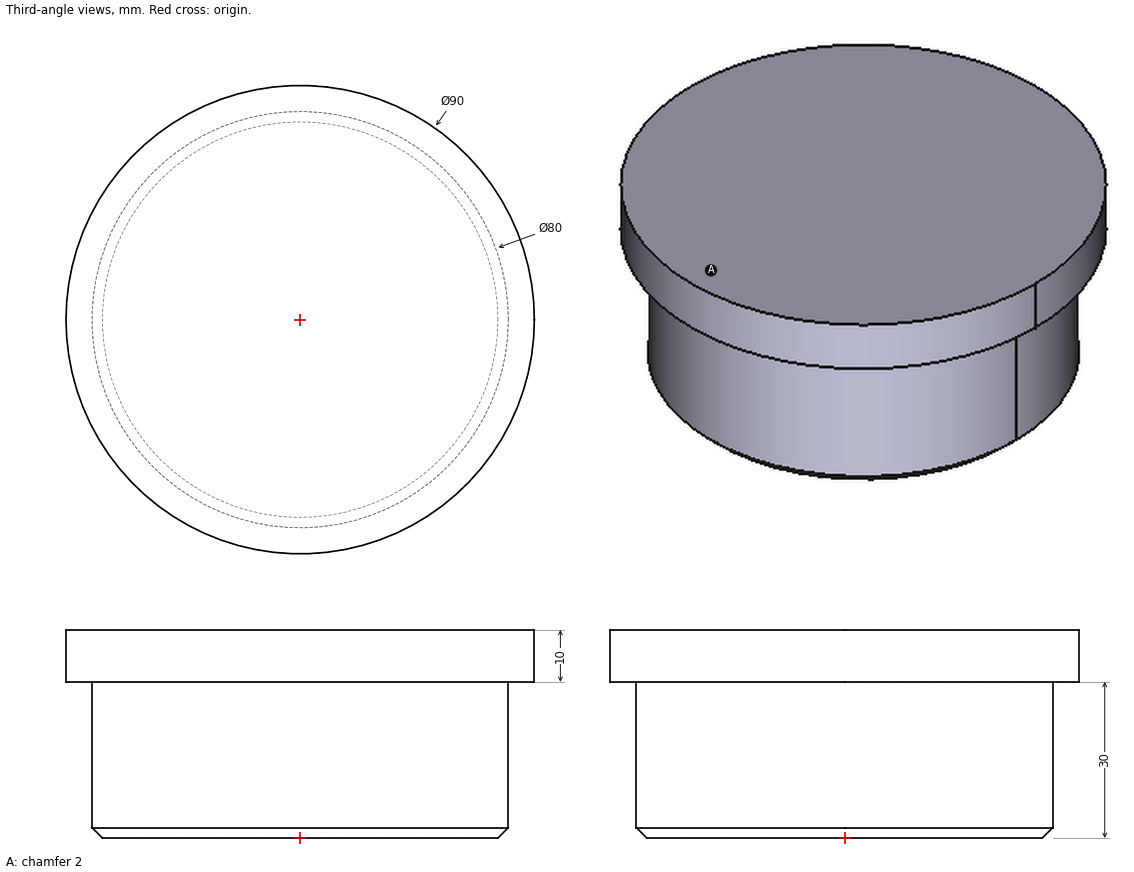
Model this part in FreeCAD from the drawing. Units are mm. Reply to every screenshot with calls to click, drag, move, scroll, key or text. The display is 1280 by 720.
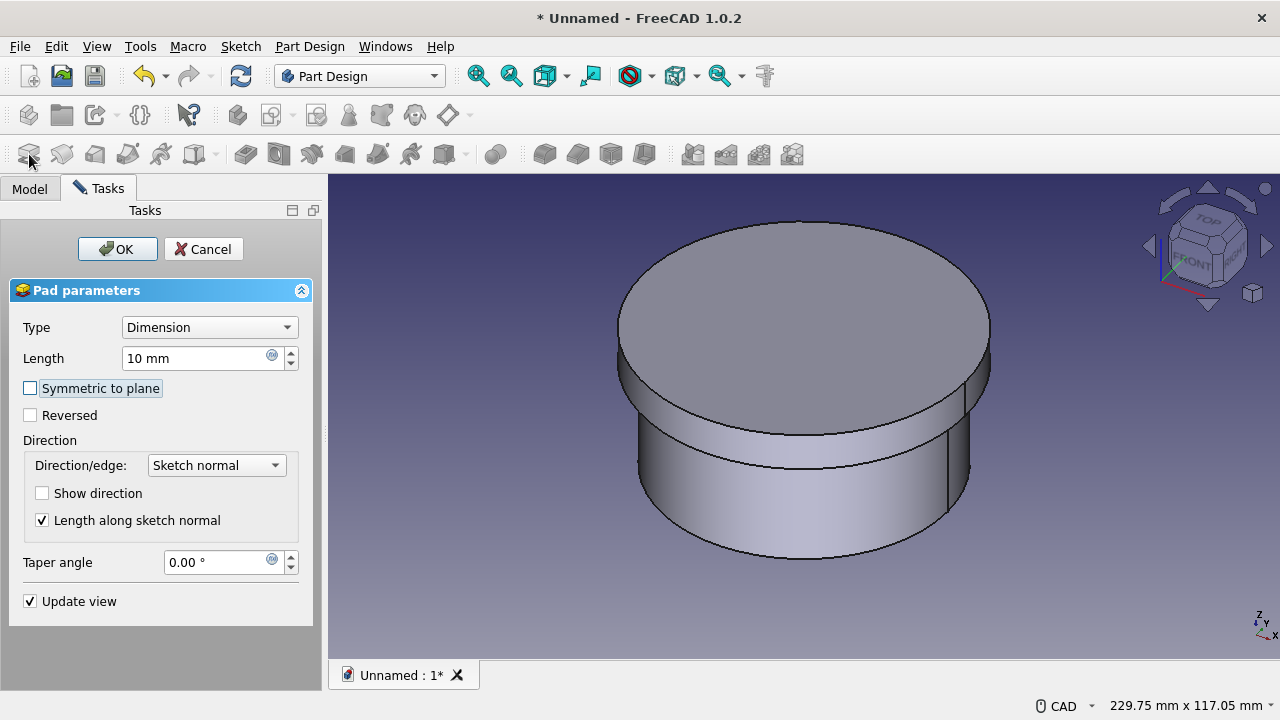
click(118, 249)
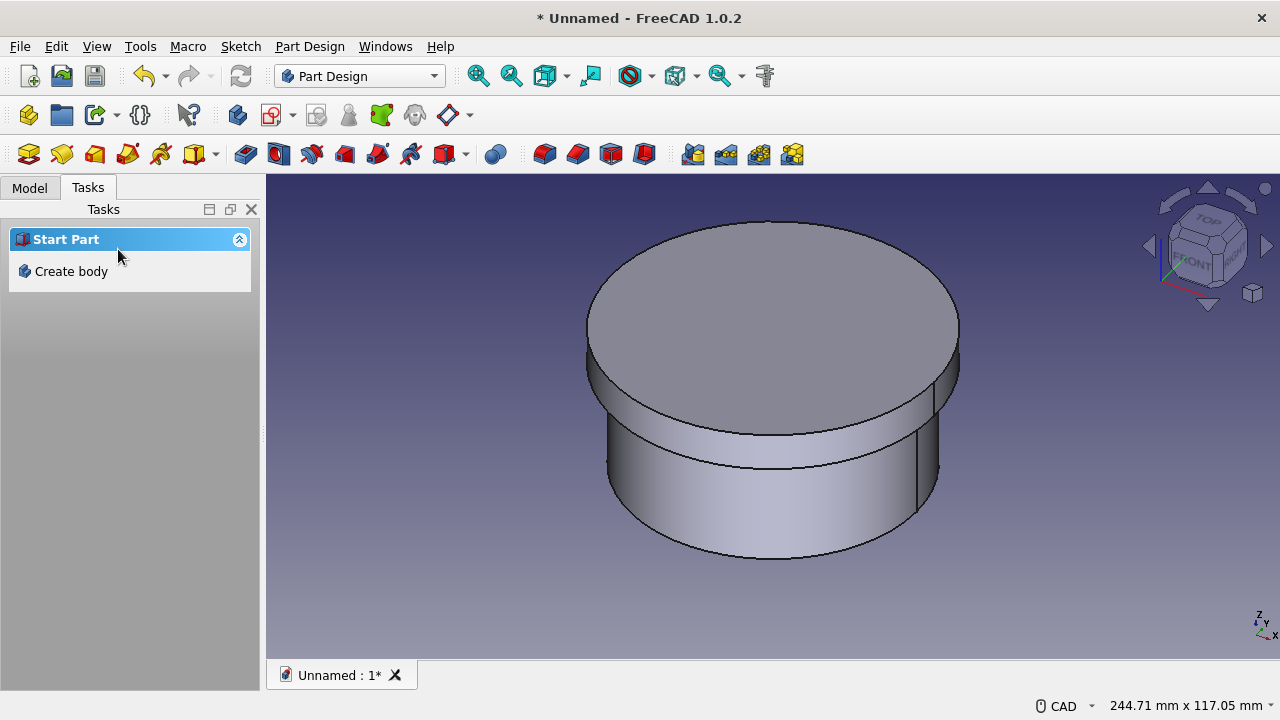
key(0)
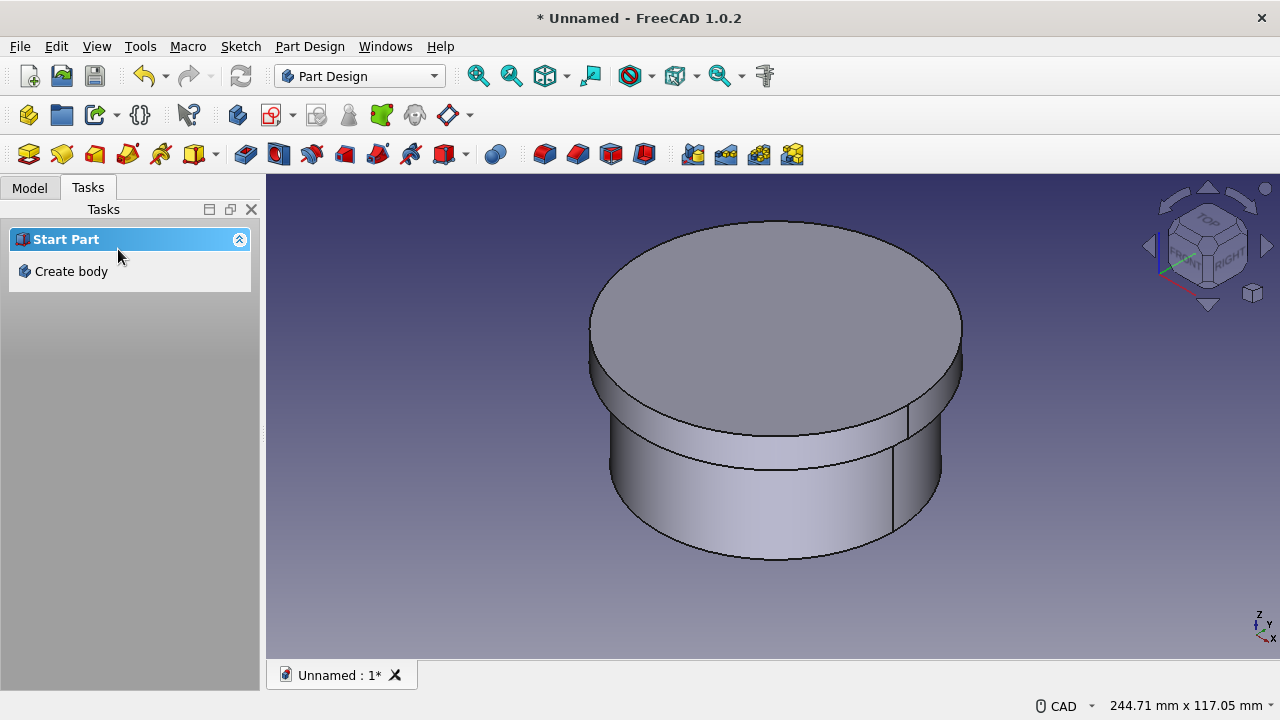
key(2)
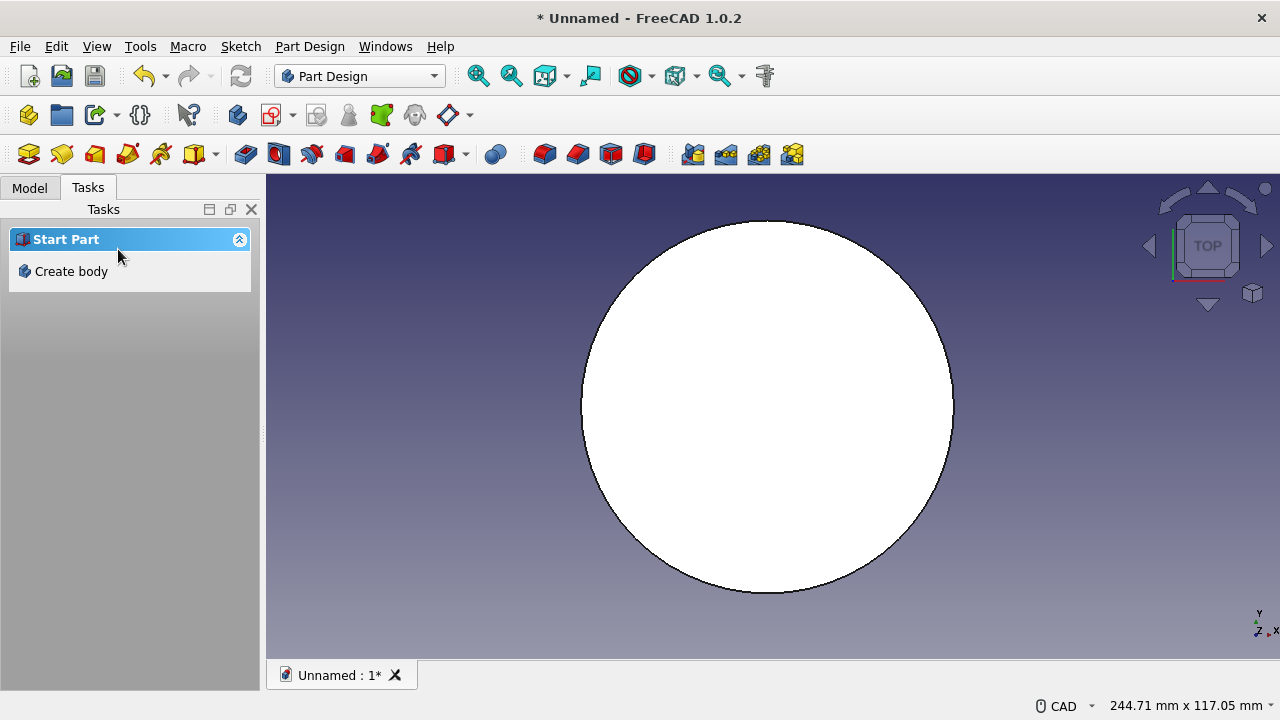
key(1)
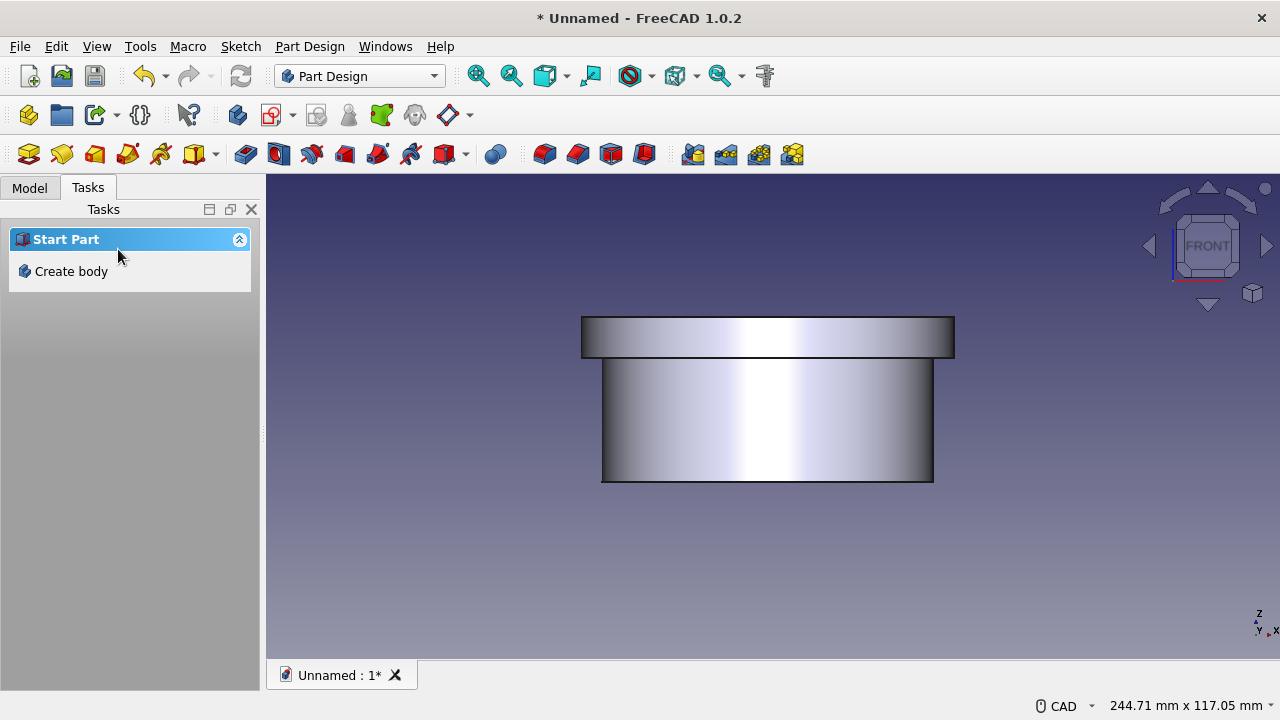
click(479, 76)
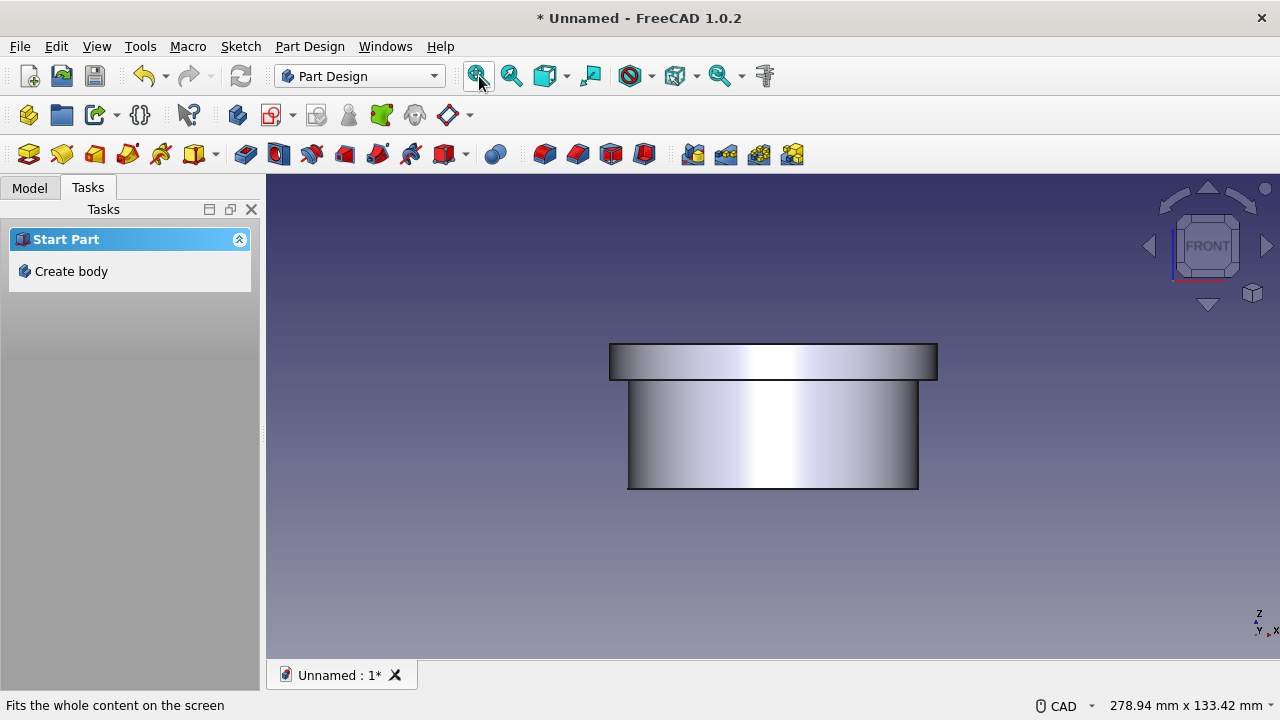
click(655, 488)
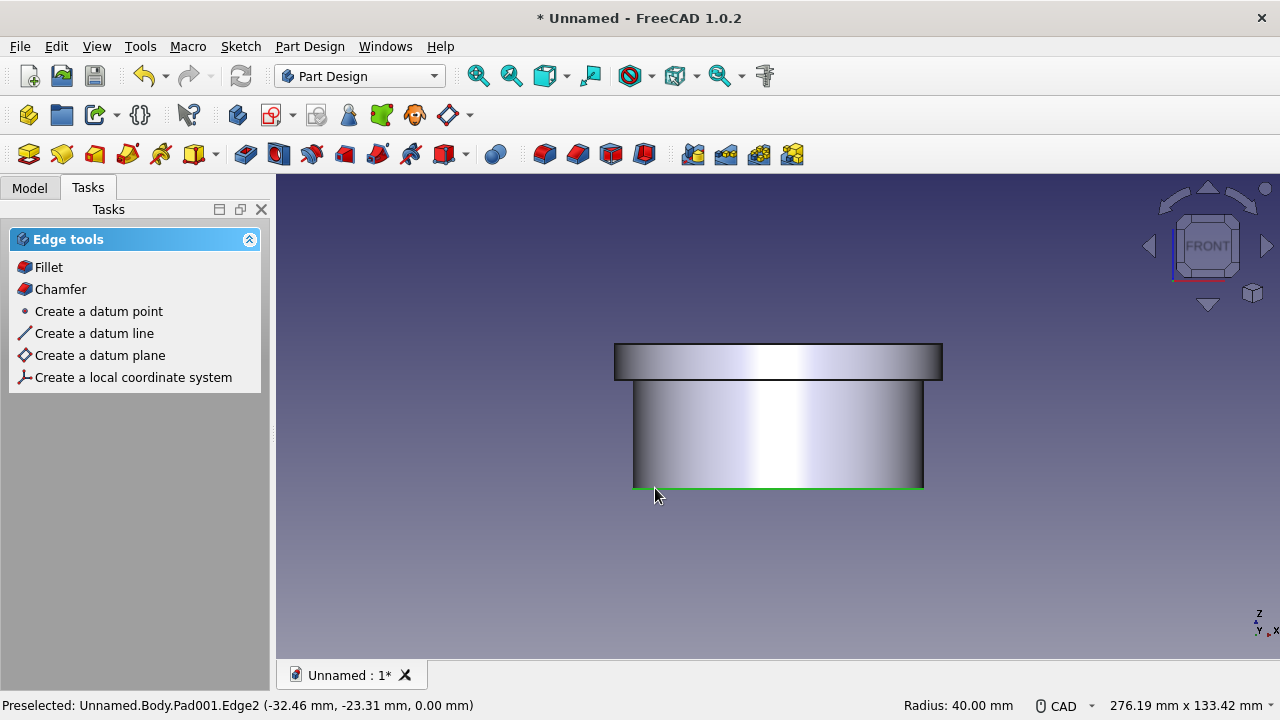
click(578, 154)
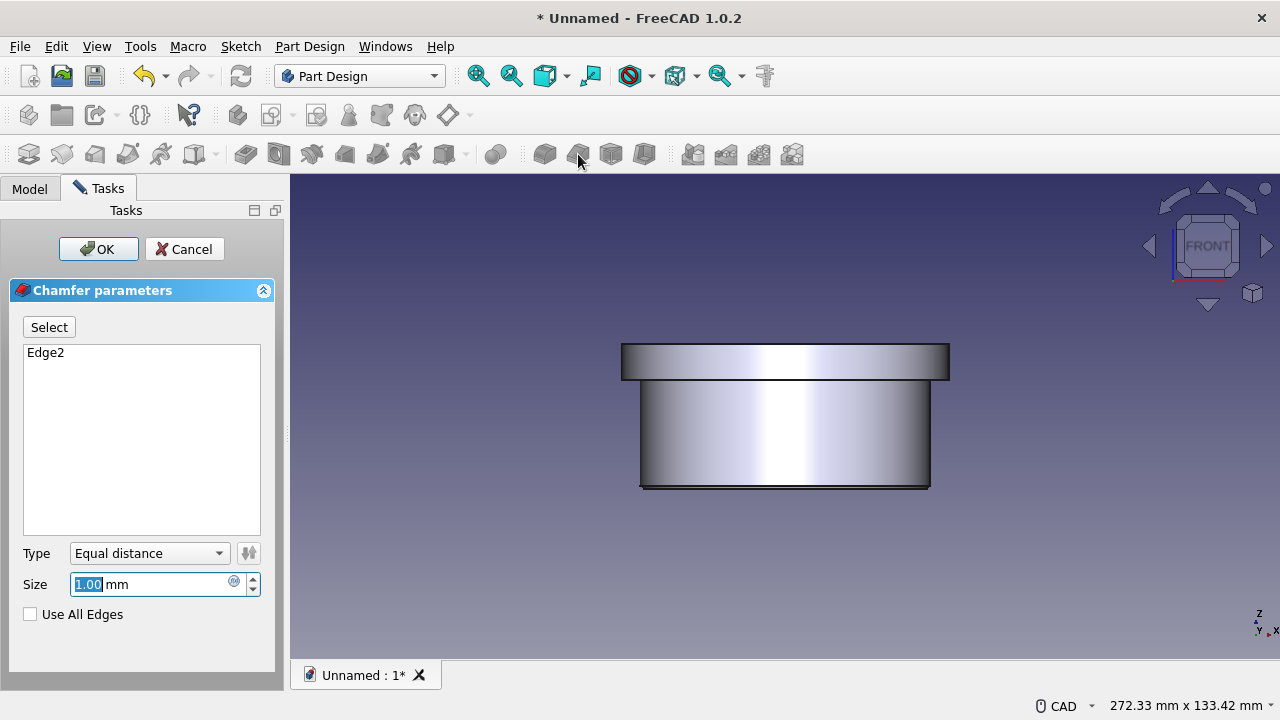
text(2)
key(Tab)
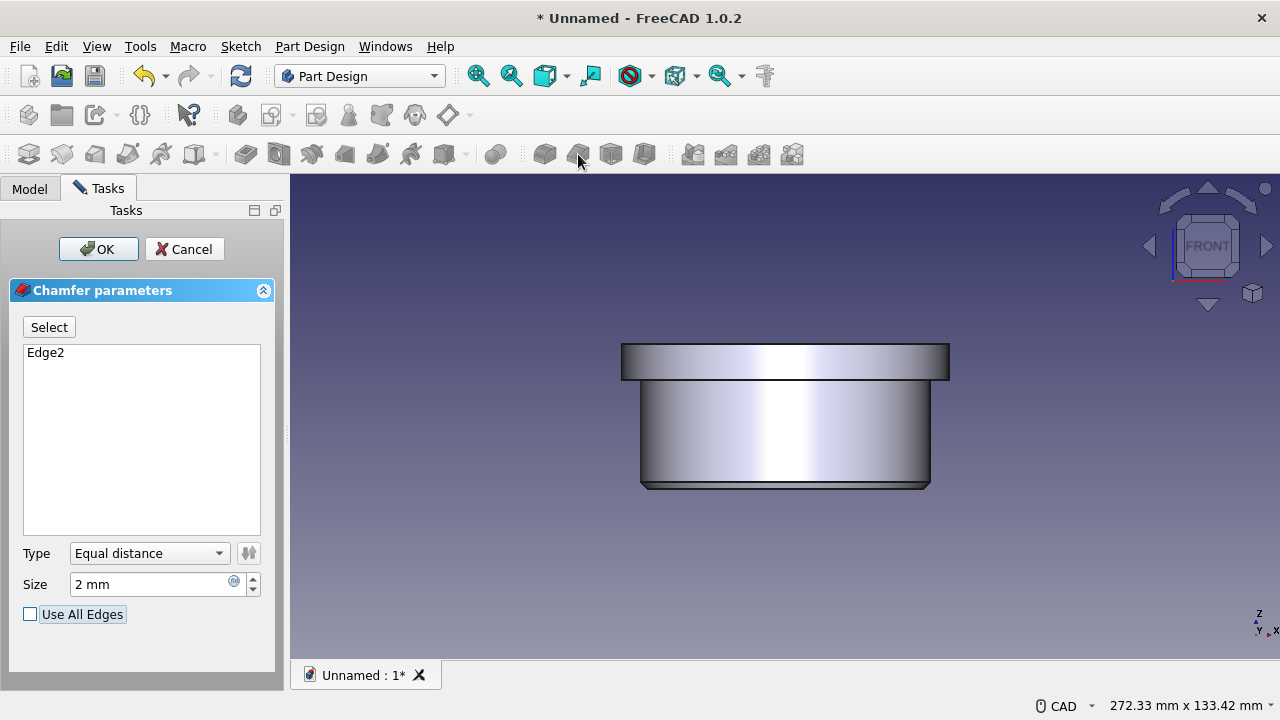
click(99, 249)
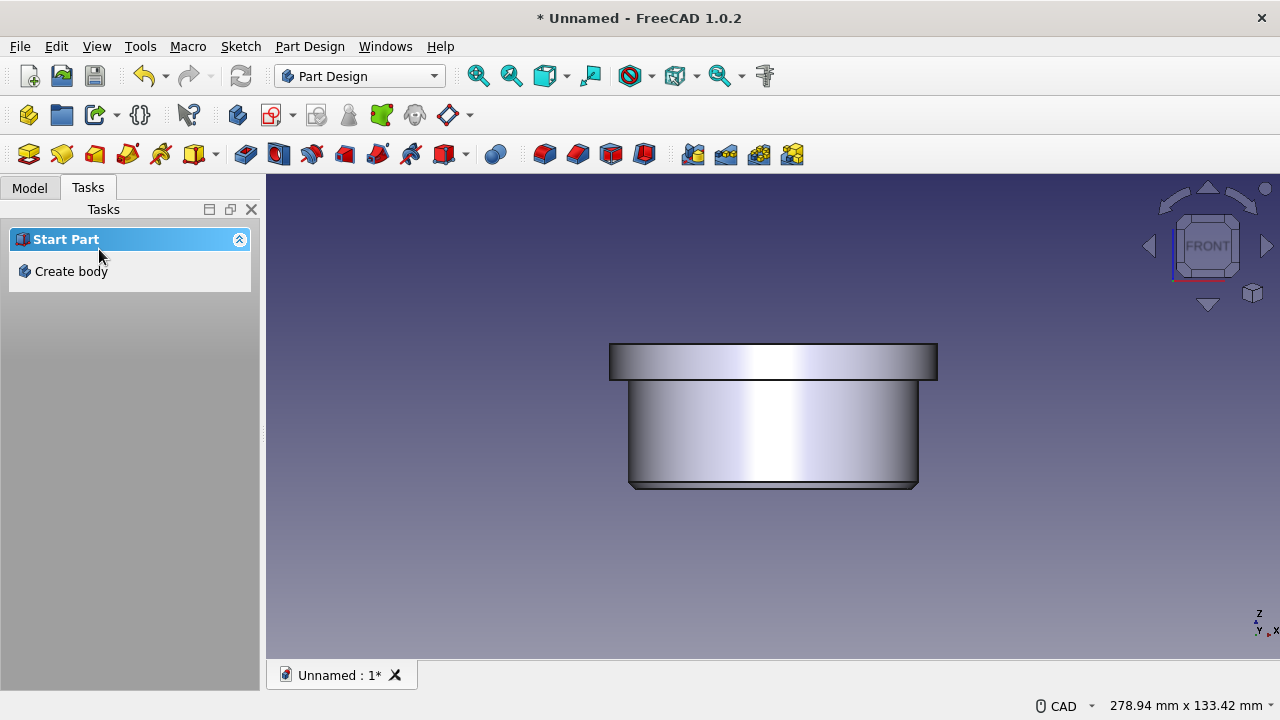
key(0)